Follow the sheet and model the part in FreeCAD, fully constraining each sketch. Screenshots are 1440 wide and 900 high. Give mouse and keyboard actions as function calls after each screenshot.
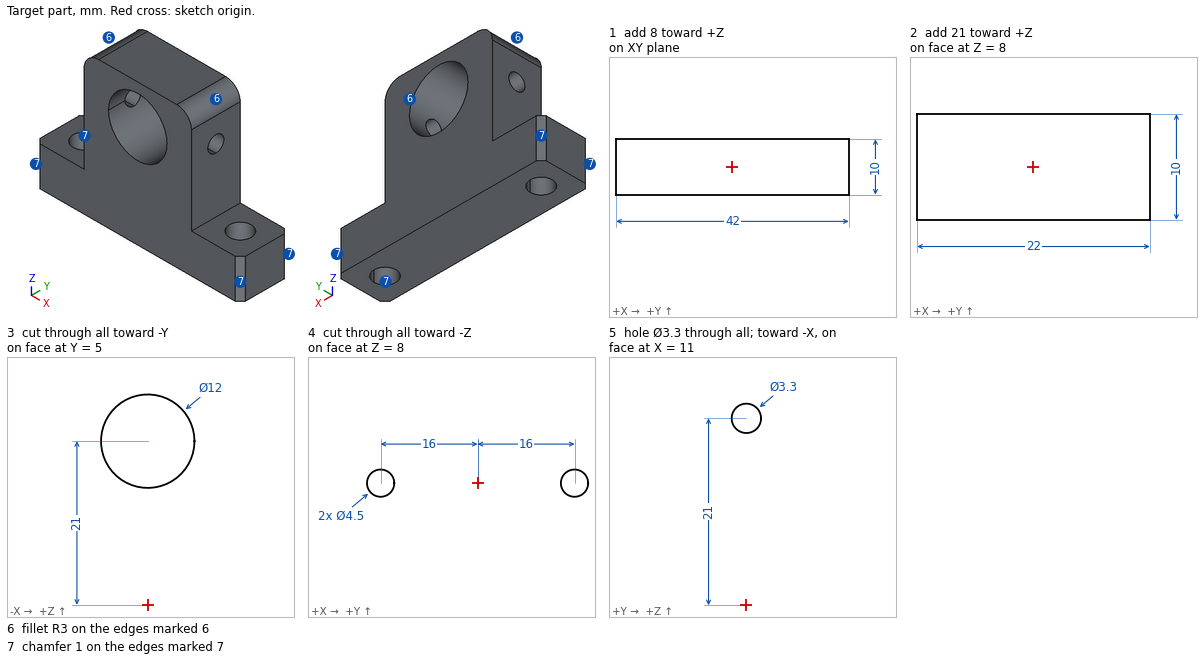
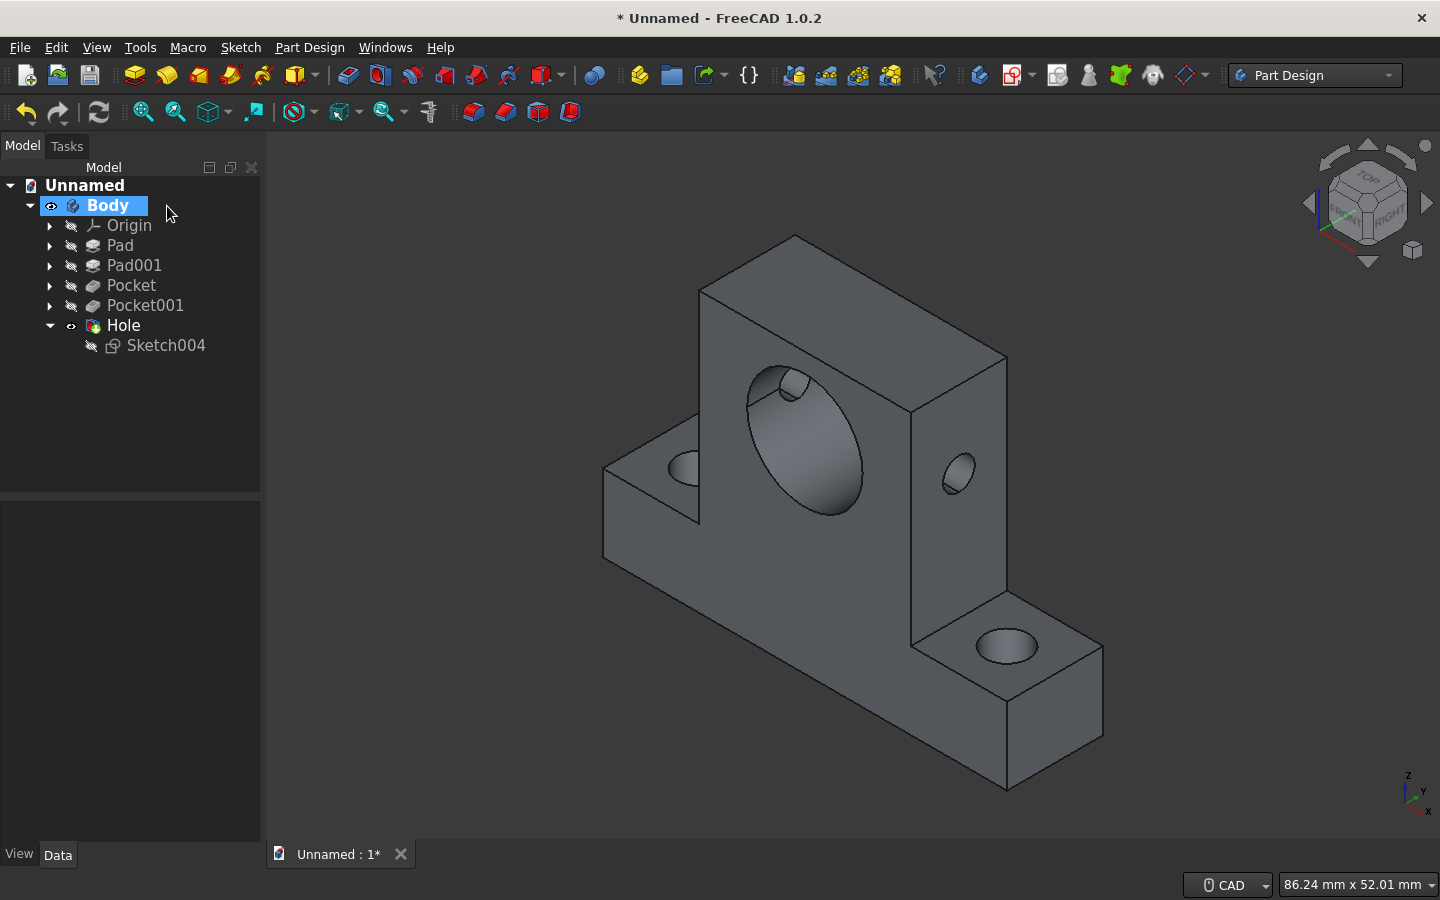
click(959, 384)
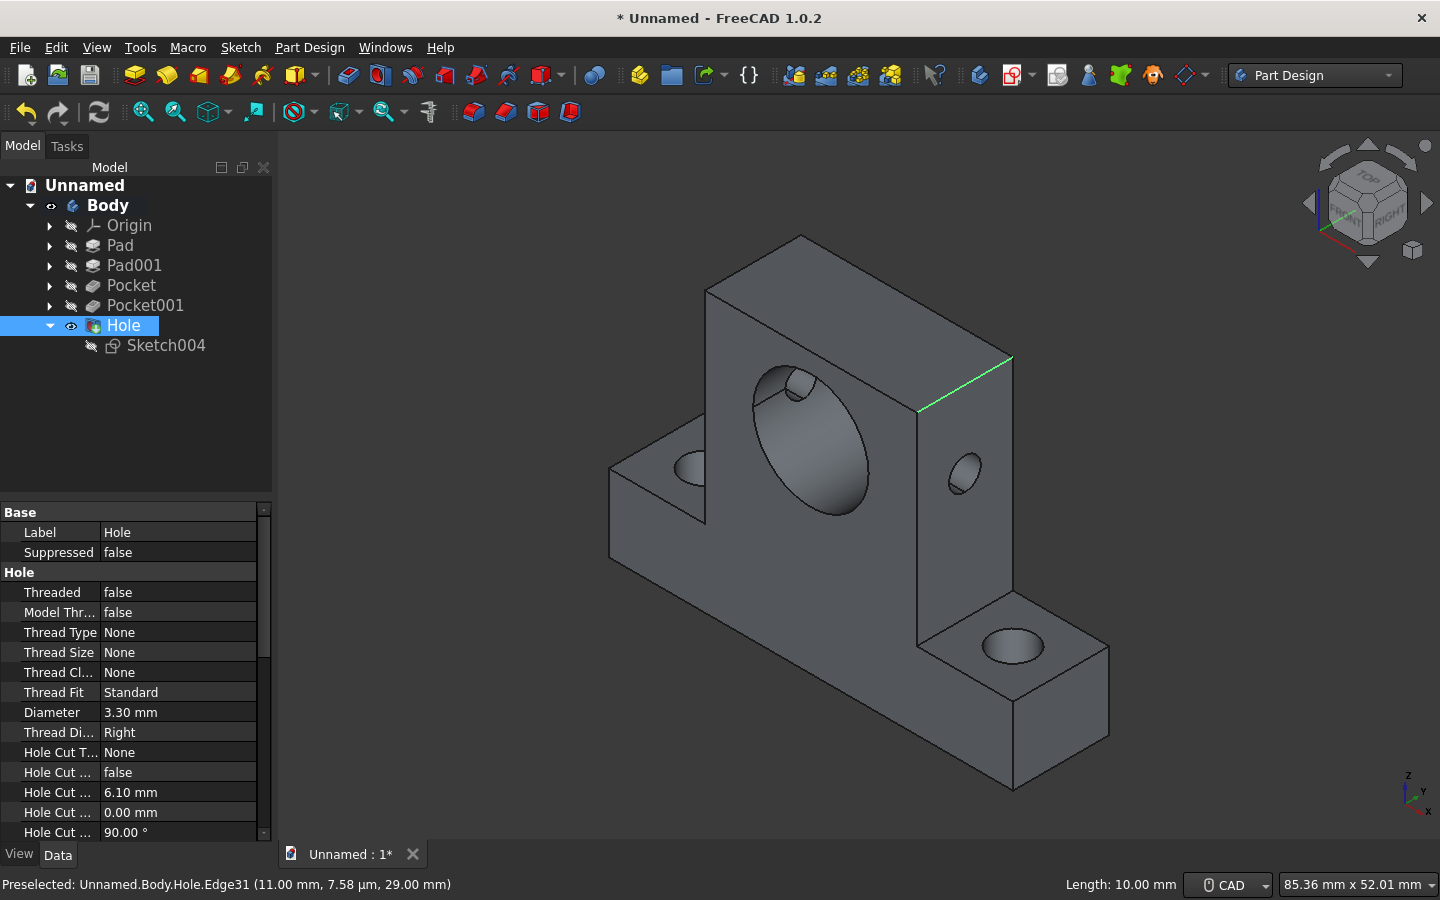
key(2)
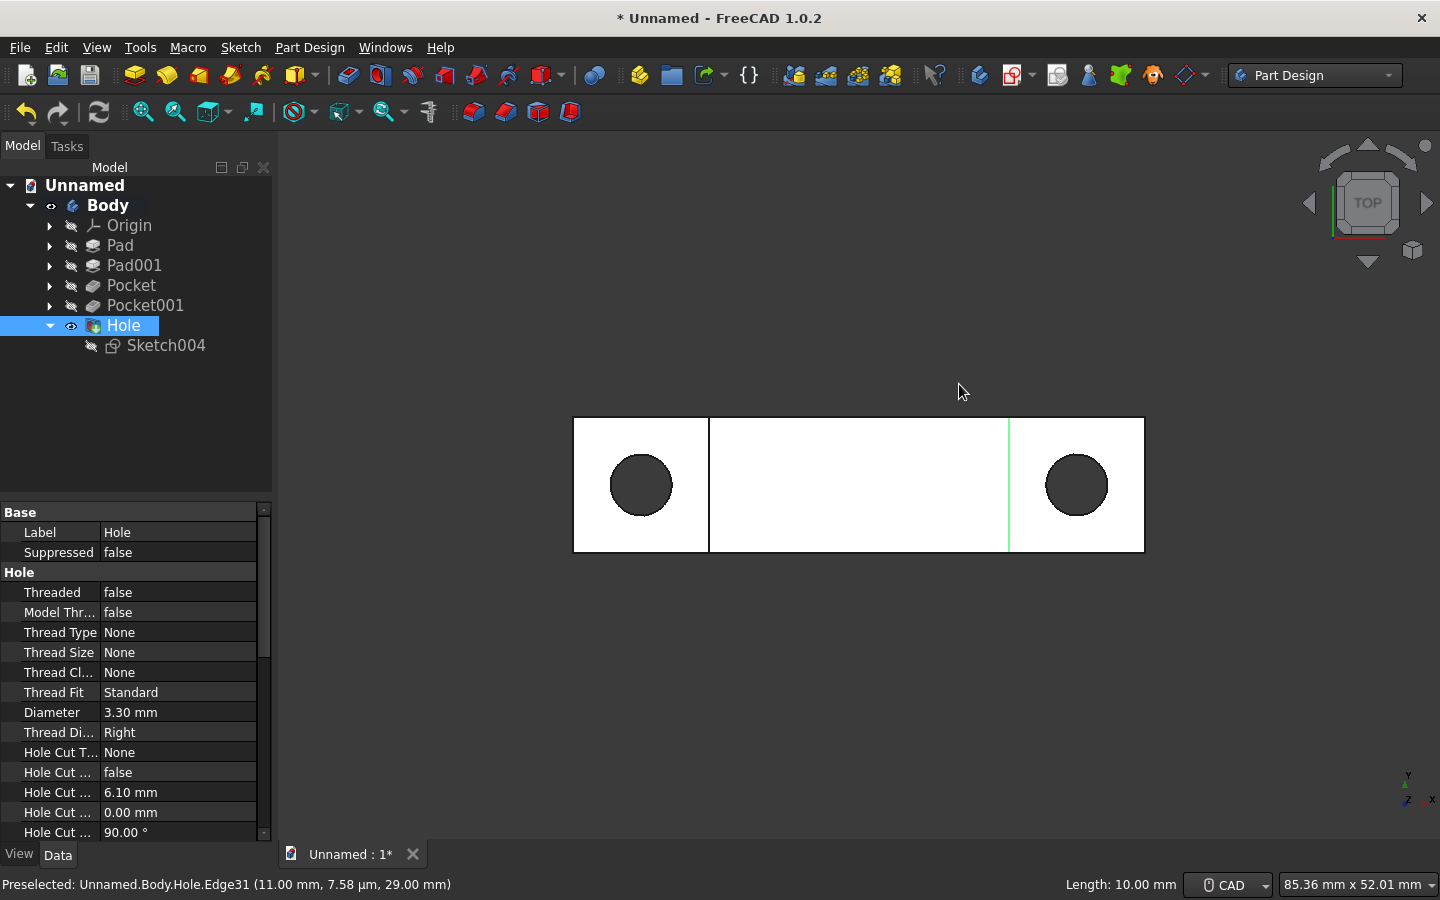
click(709, 484, ctrl)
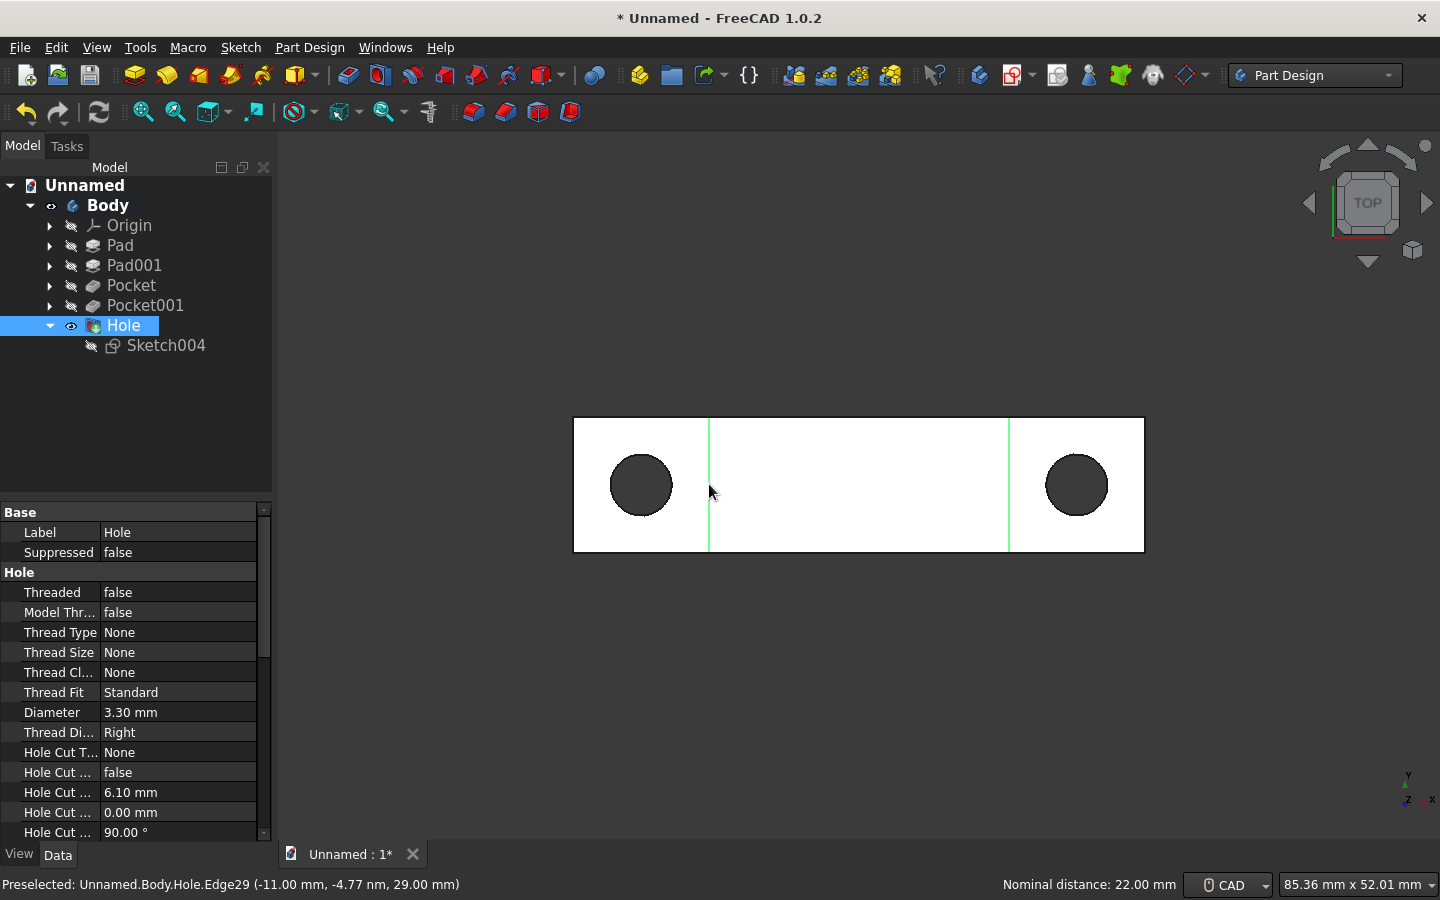
click(474, 112)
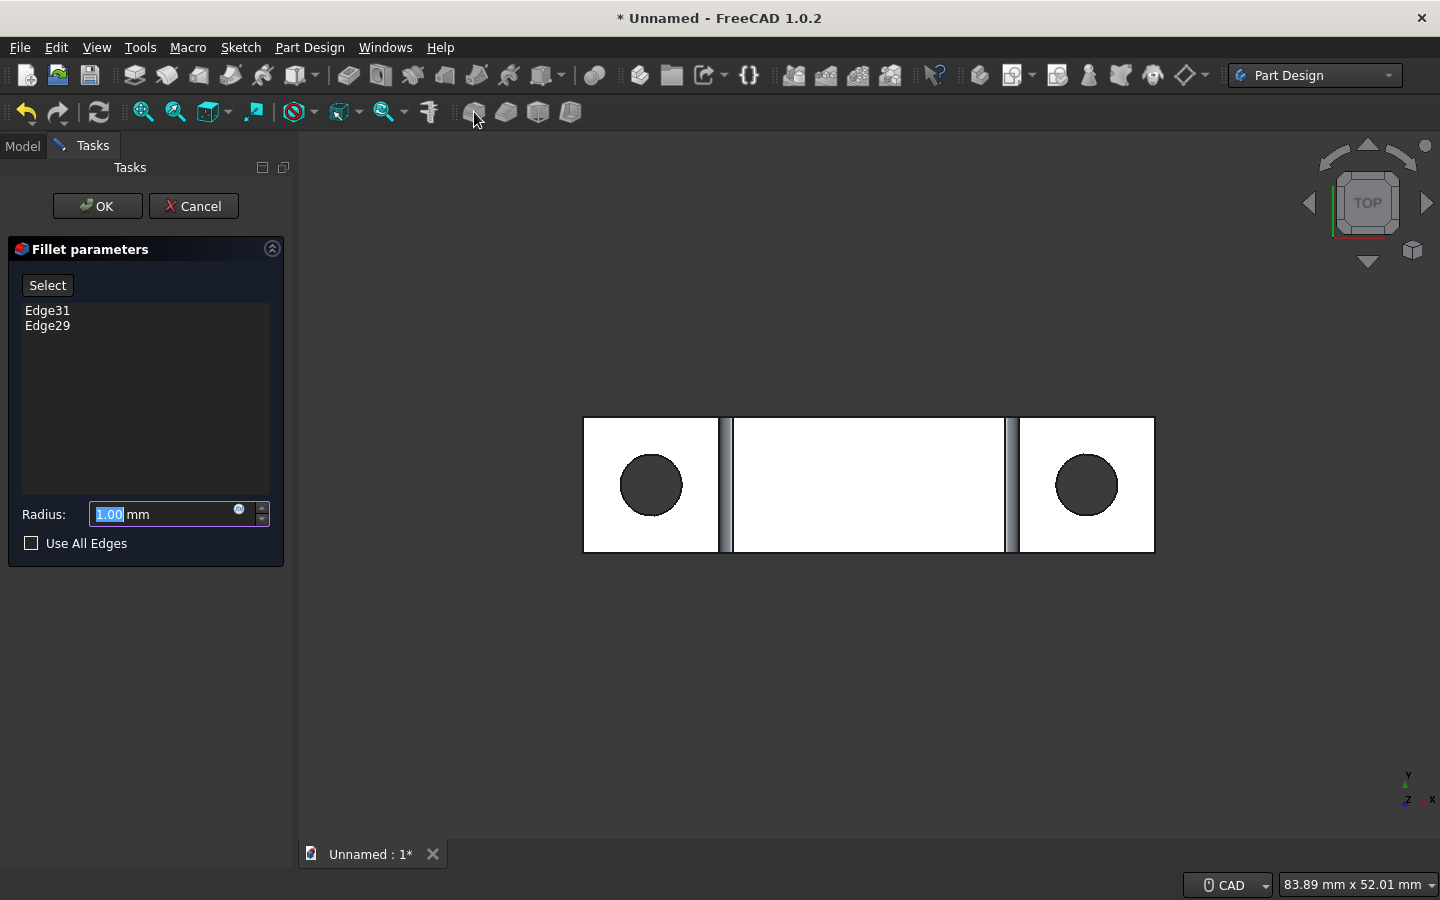
text(3)
key(Tab)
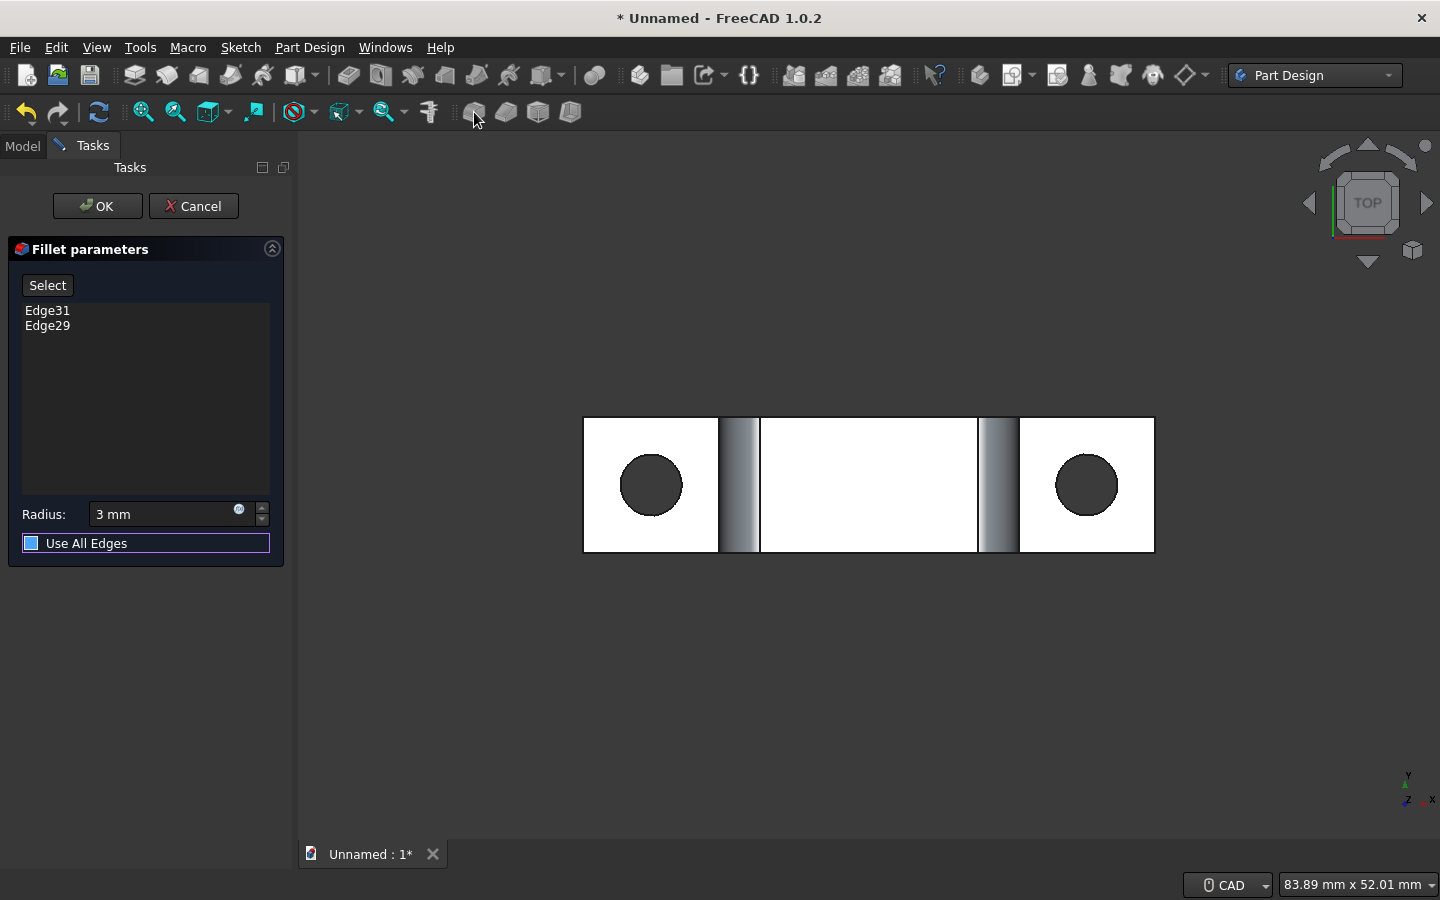
click(98, 206)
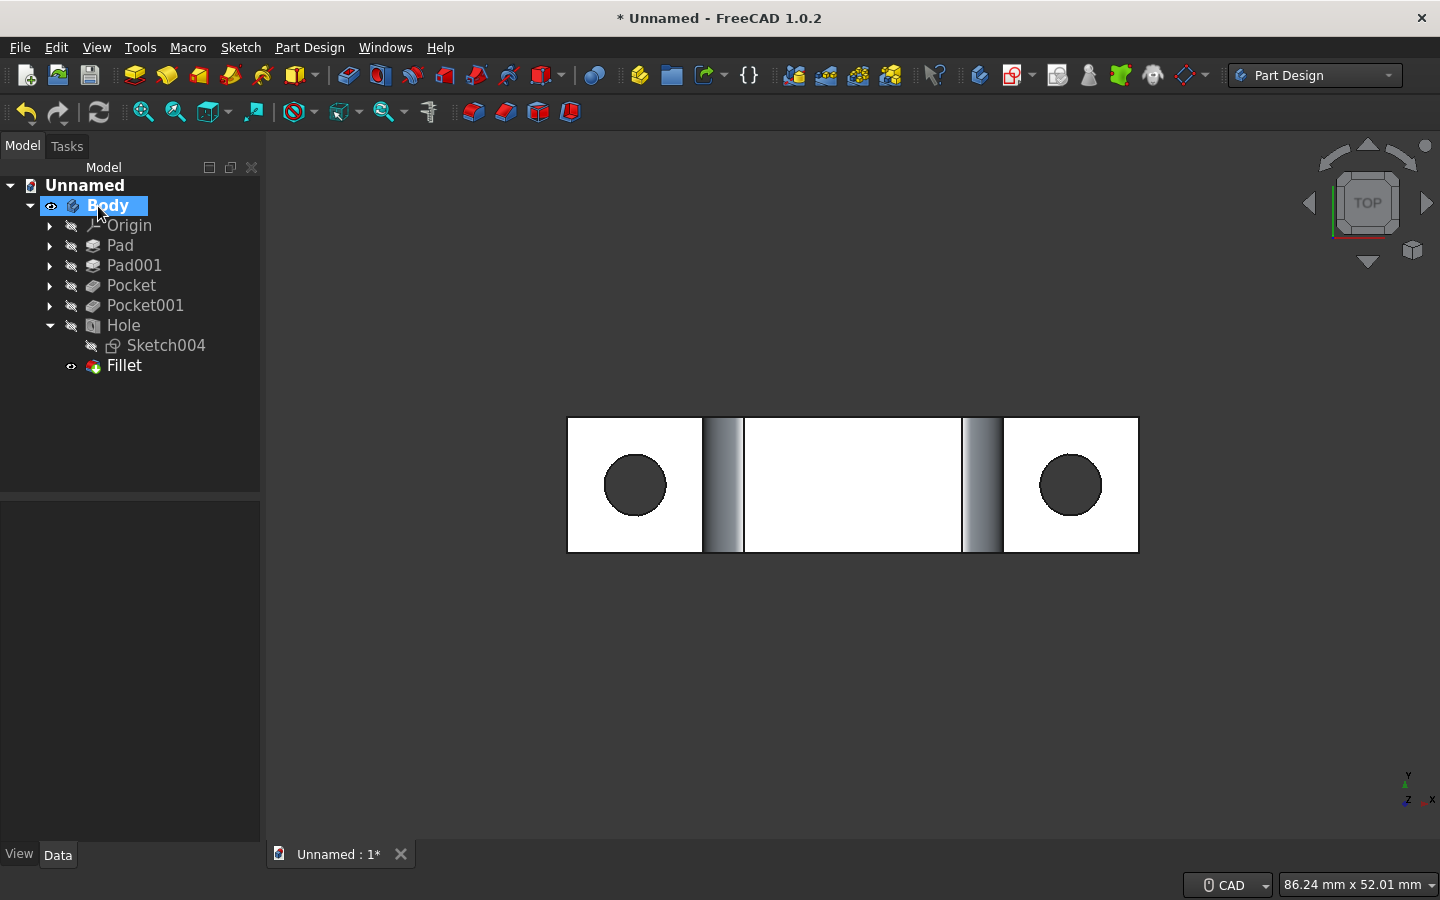
key(0)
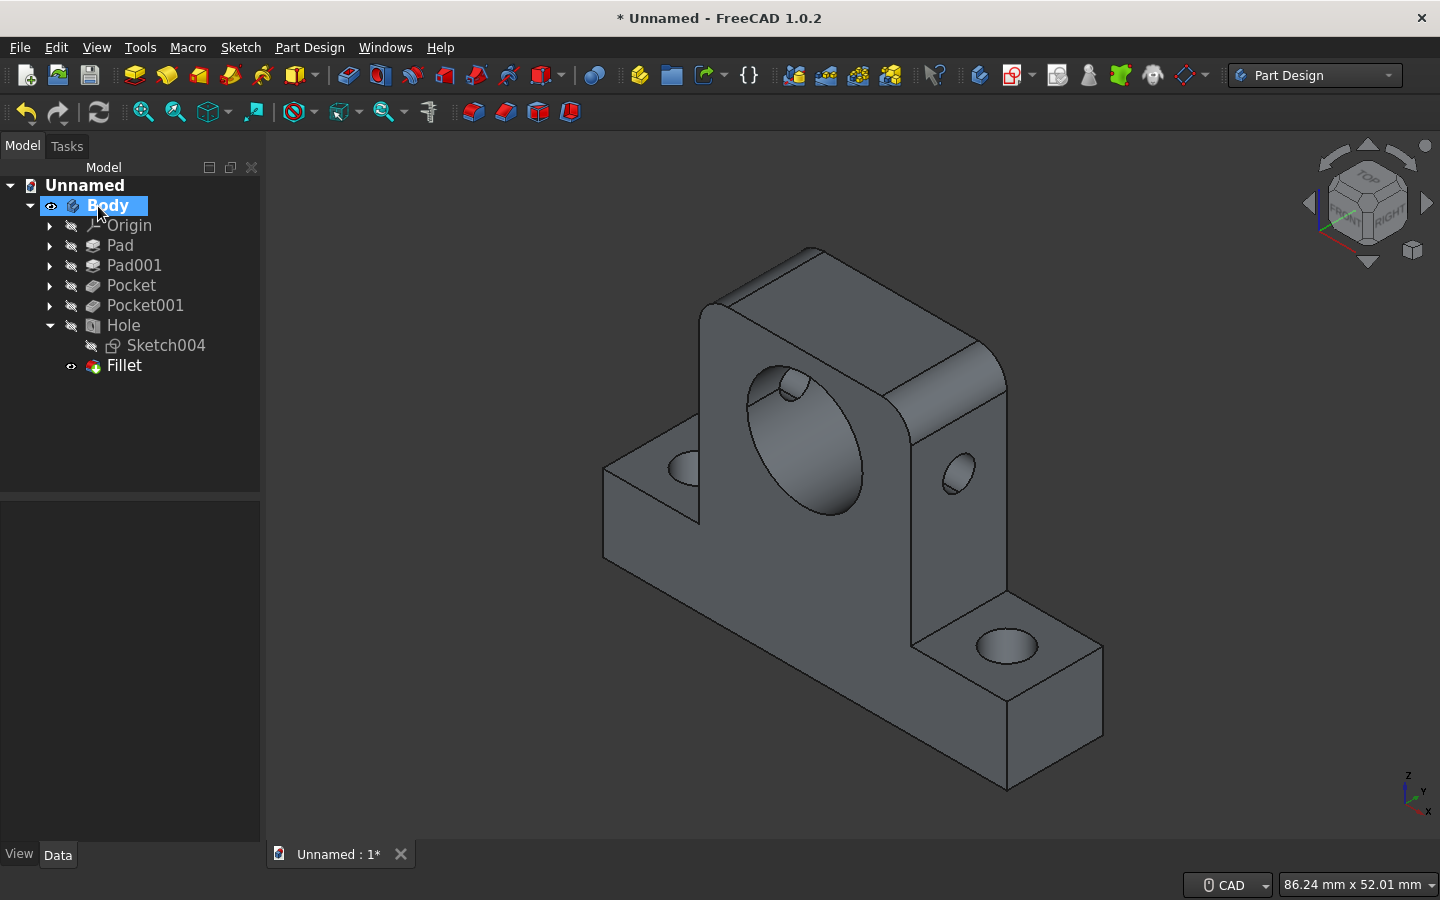
click(1007, 745)